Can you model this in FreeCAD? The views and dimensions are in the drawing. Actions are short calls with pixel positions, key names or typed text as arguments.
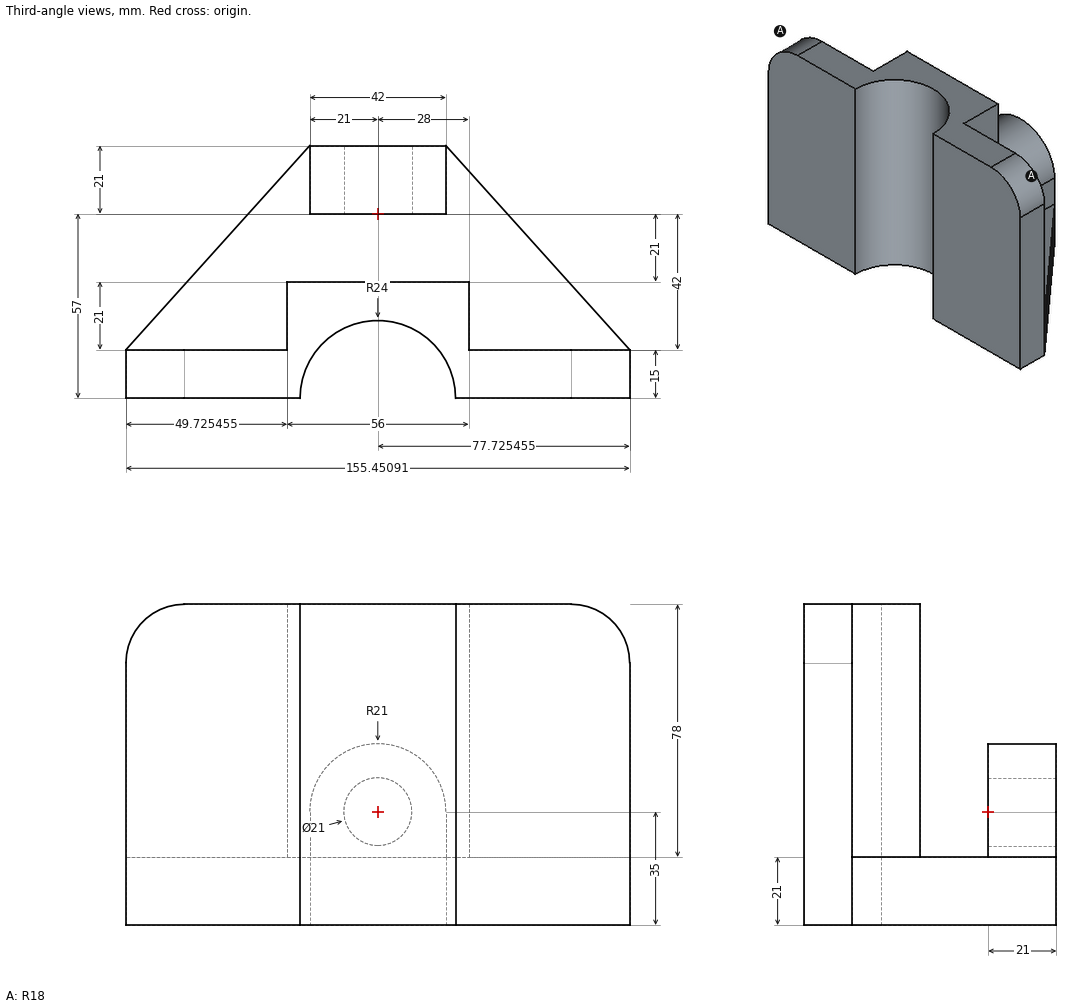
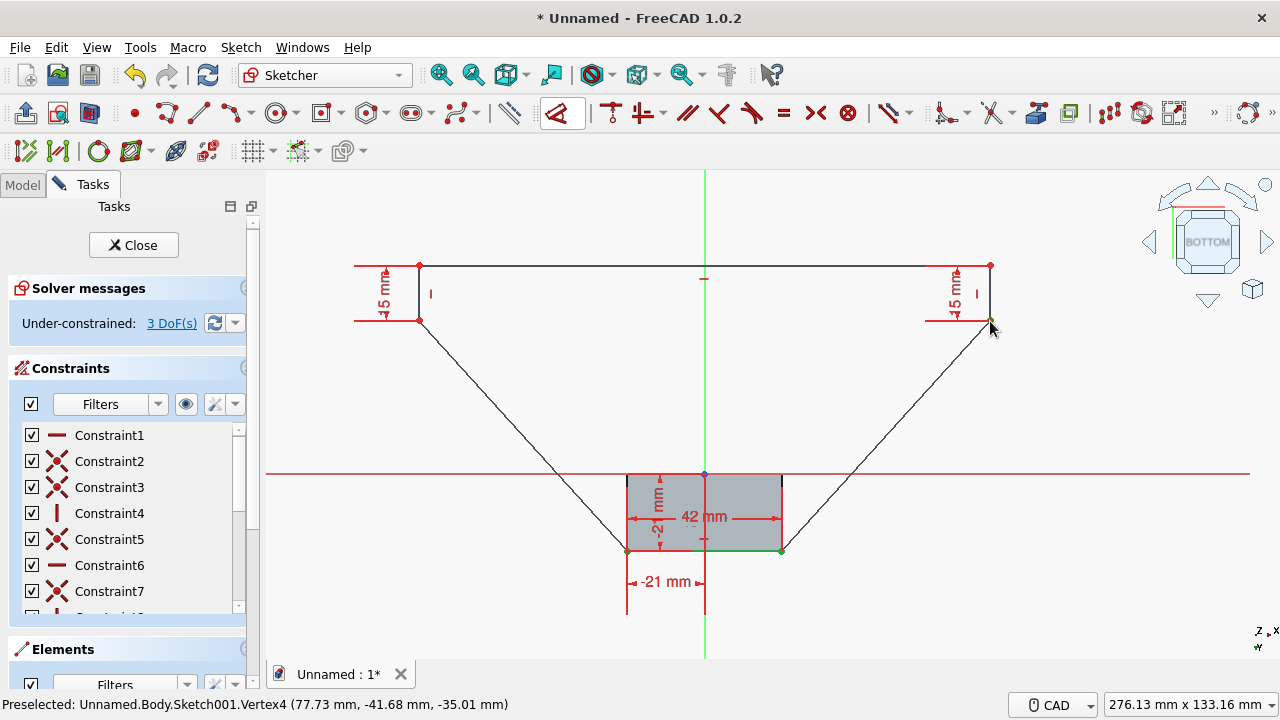
click(580, 114)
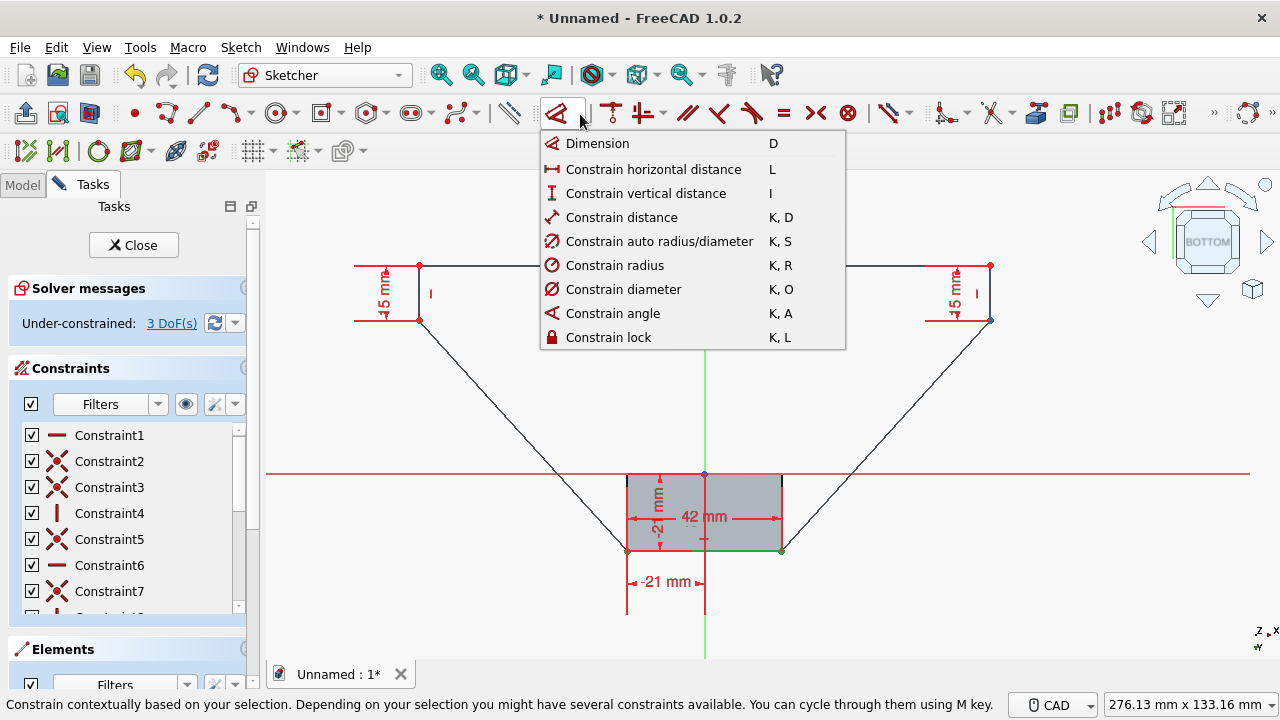
click(693, 193)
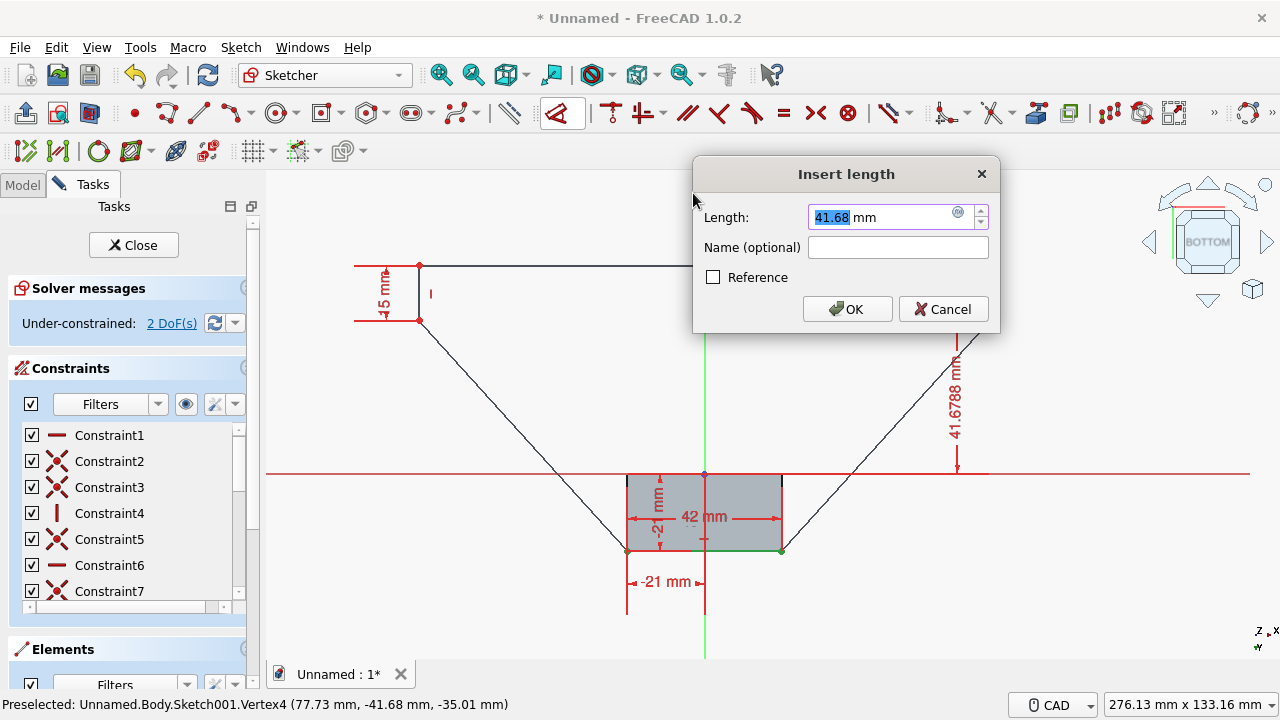
text(42)
key(Return)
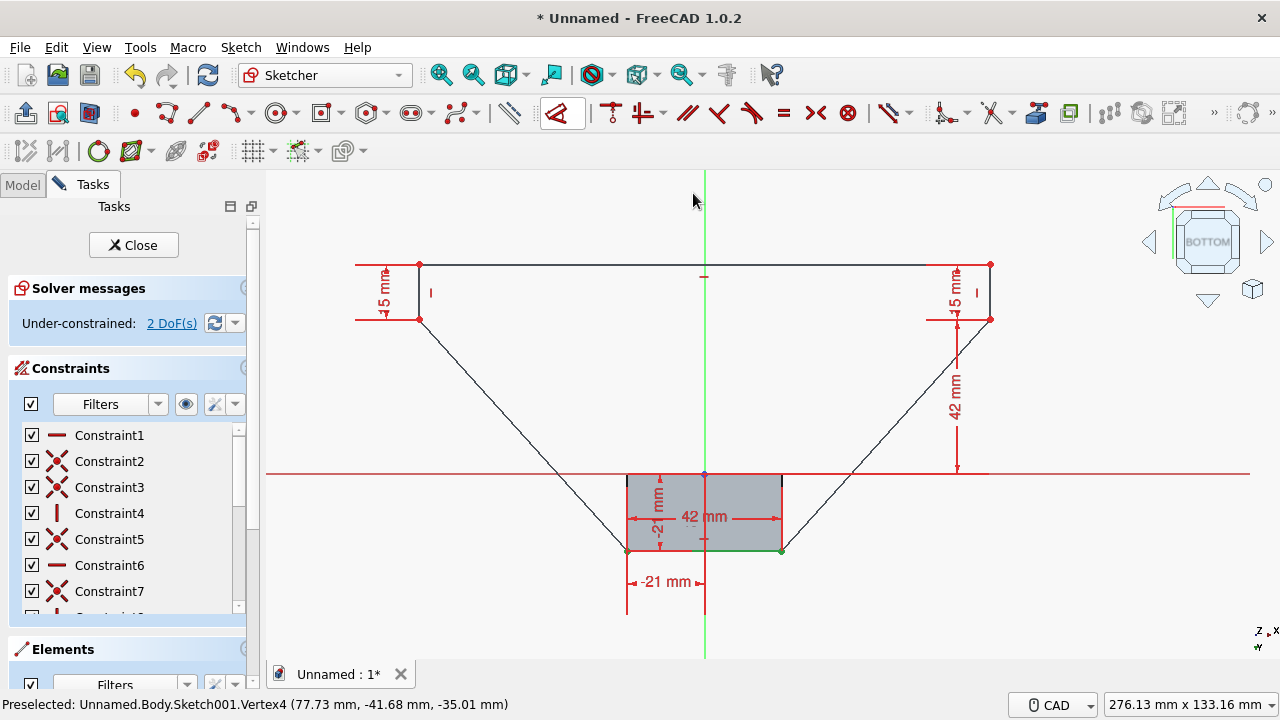
click(819, 265)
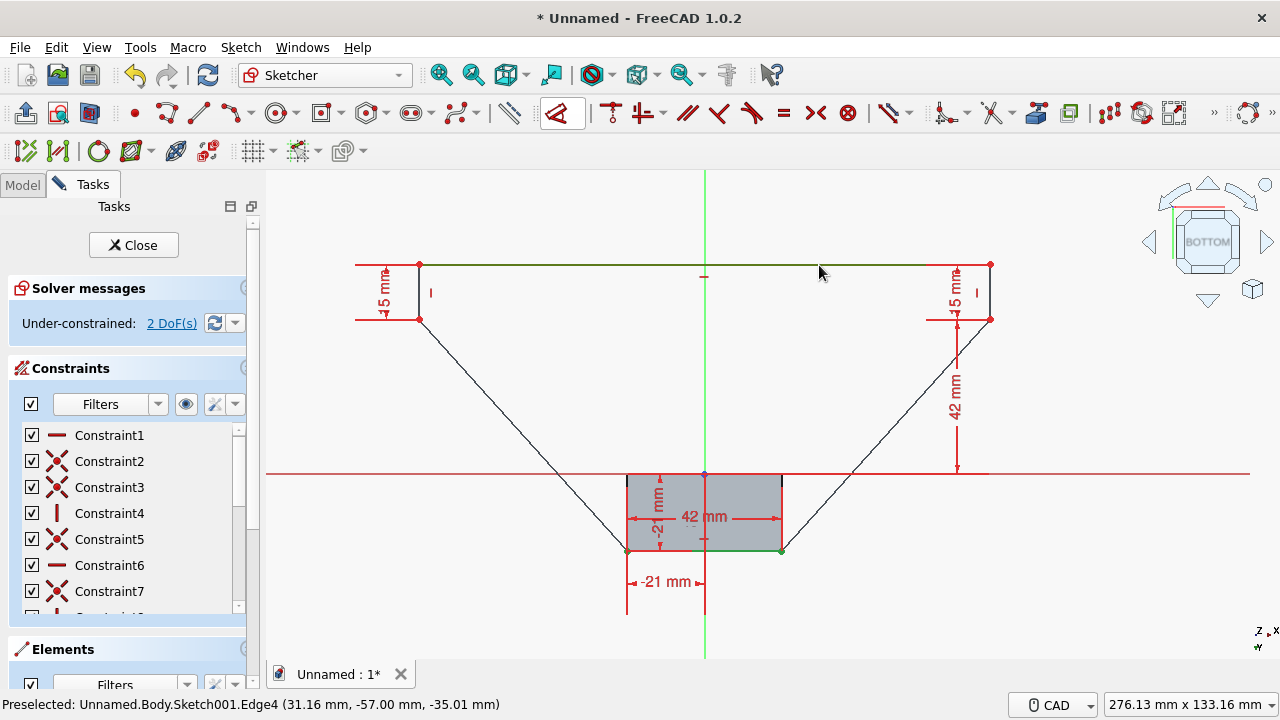
key(l)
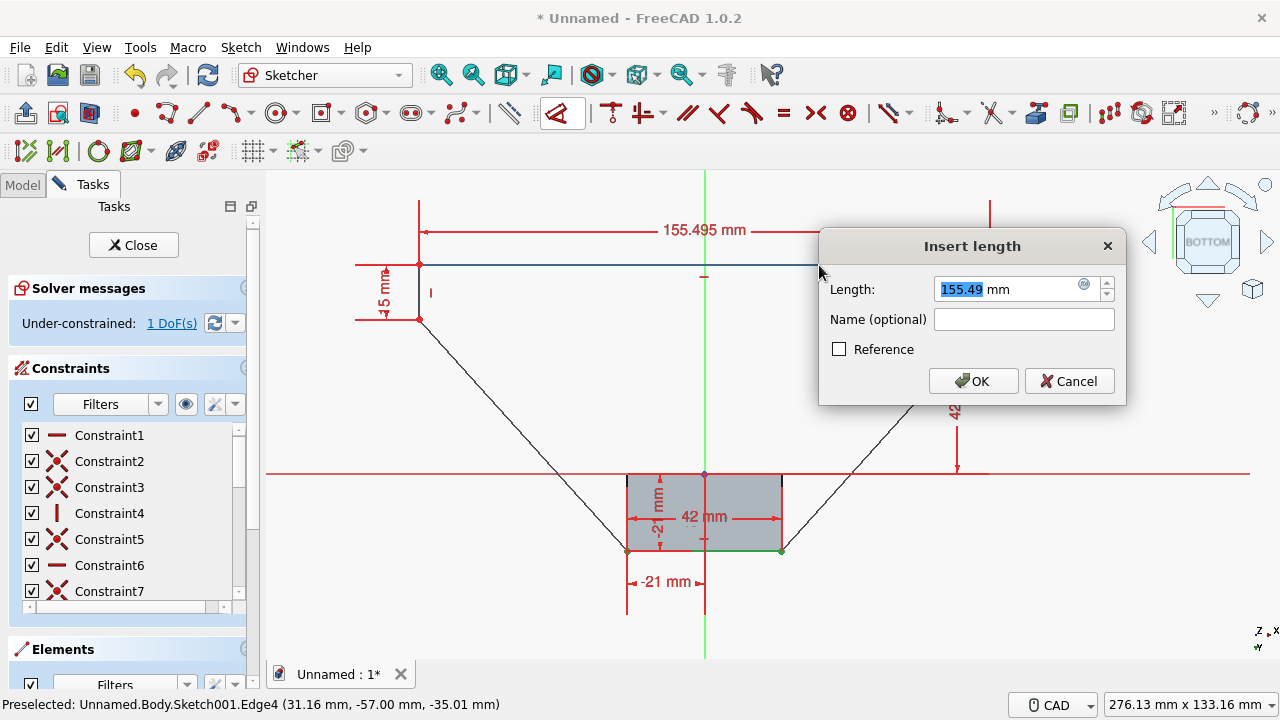
text(155.45091)
key(Return)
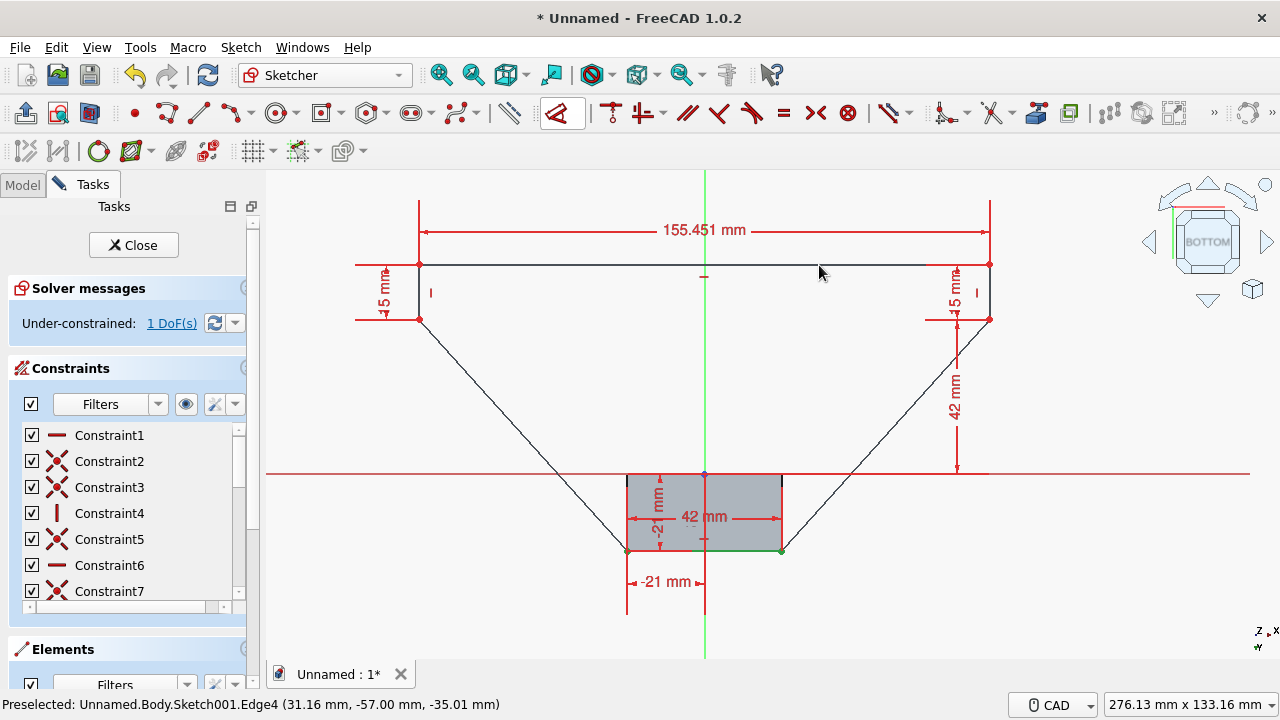
click(990, 320)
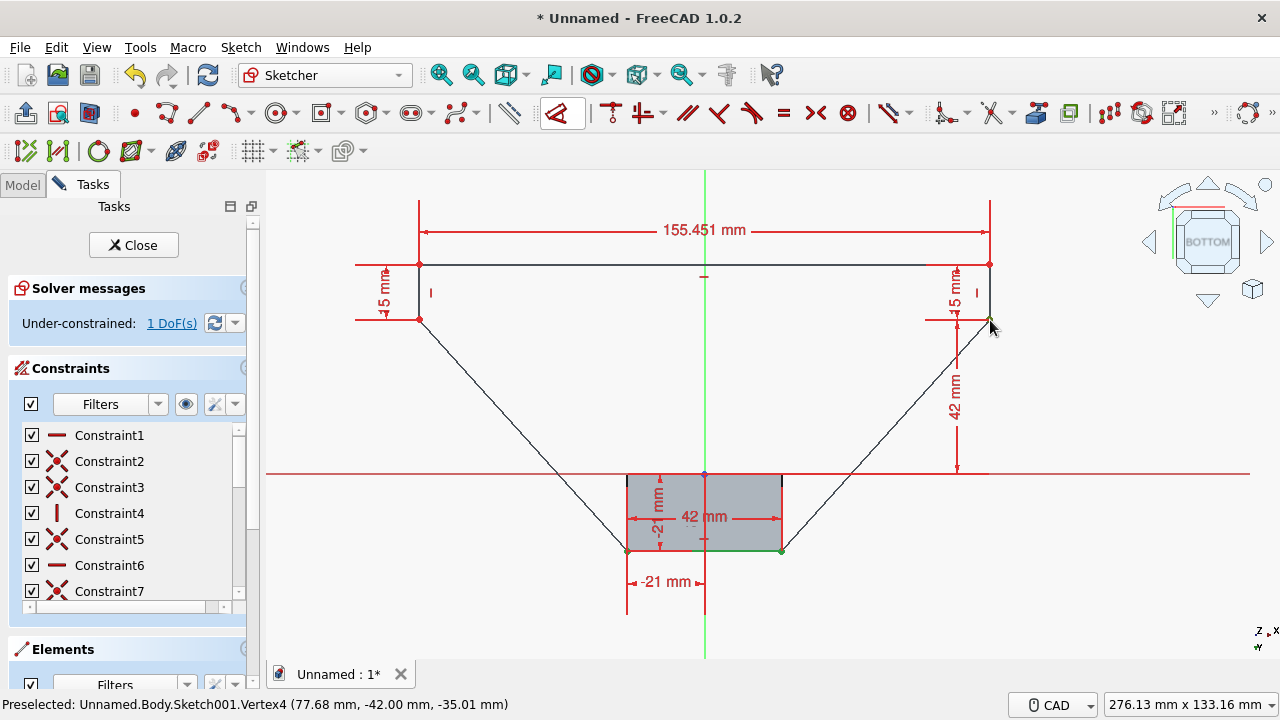
key(l)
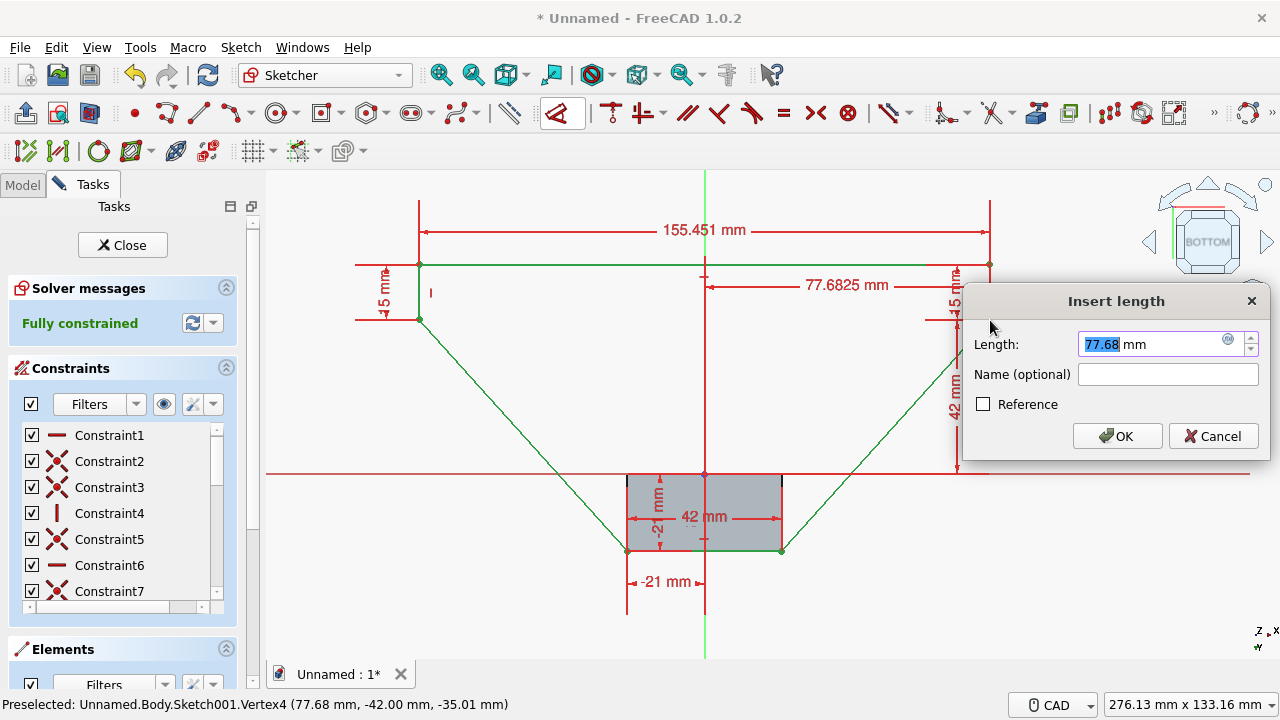
text(77.725455)
key(Return)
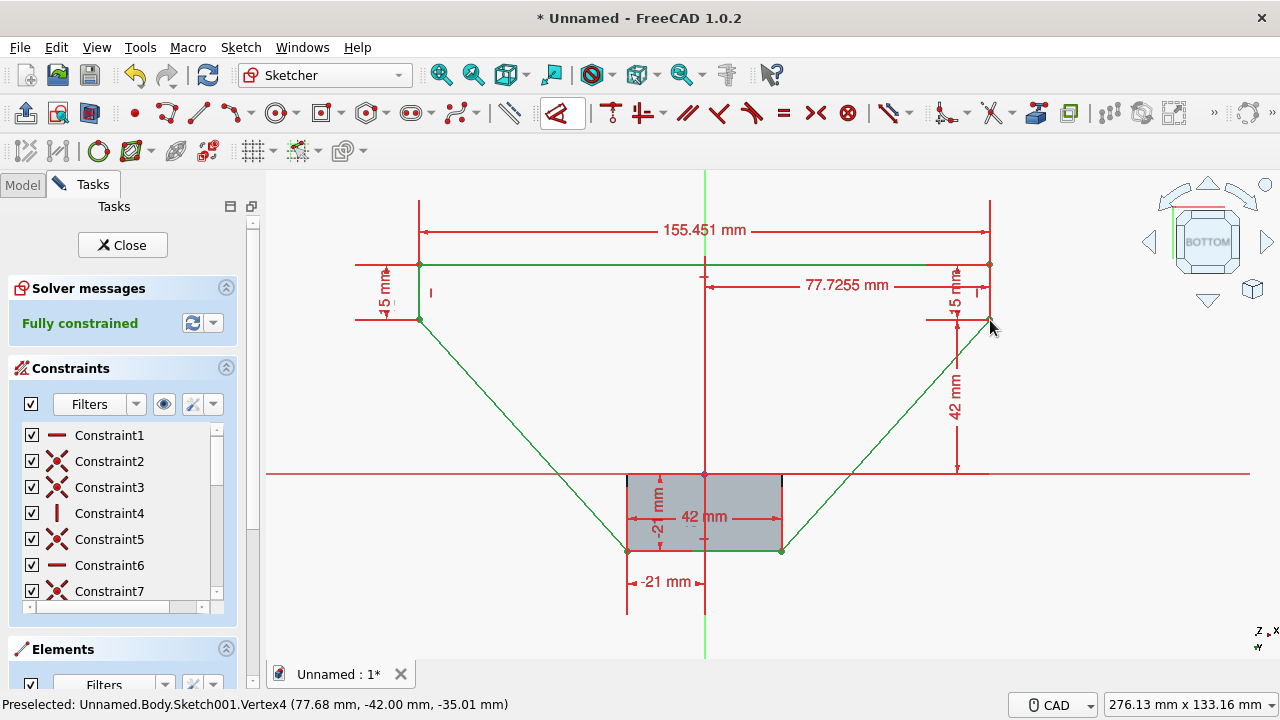
click(123, 245)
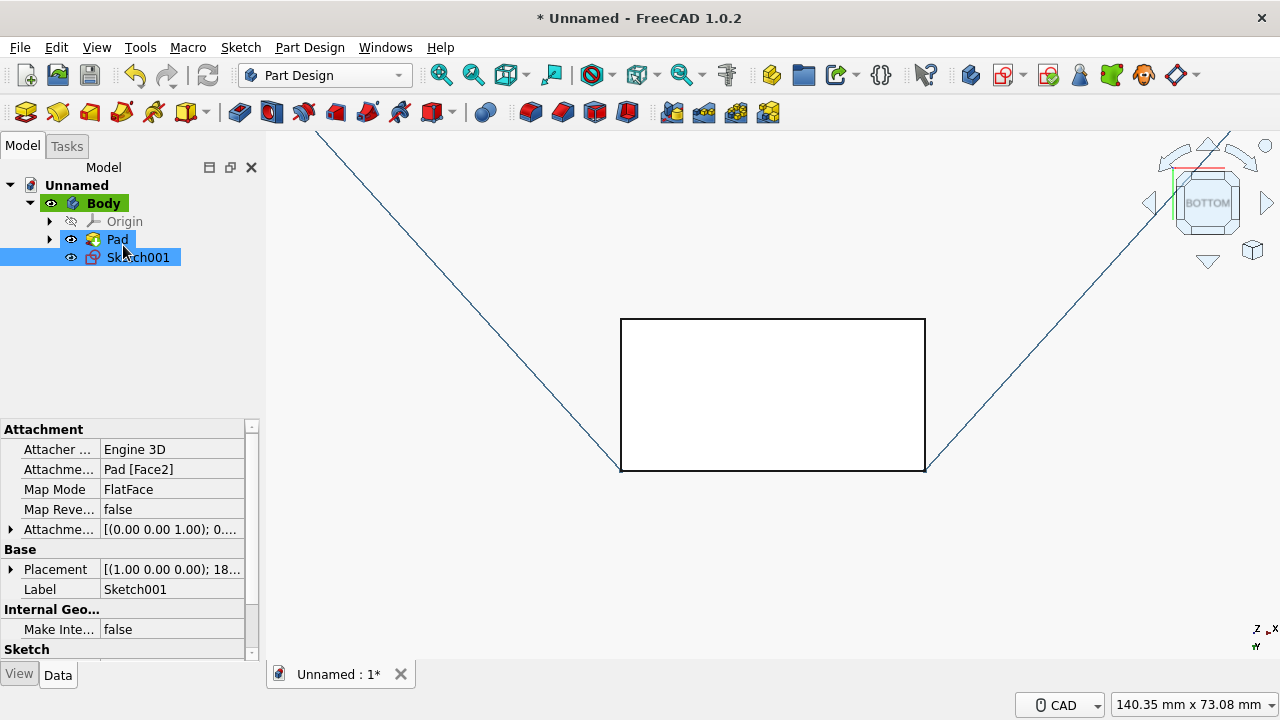
click(26, 112)